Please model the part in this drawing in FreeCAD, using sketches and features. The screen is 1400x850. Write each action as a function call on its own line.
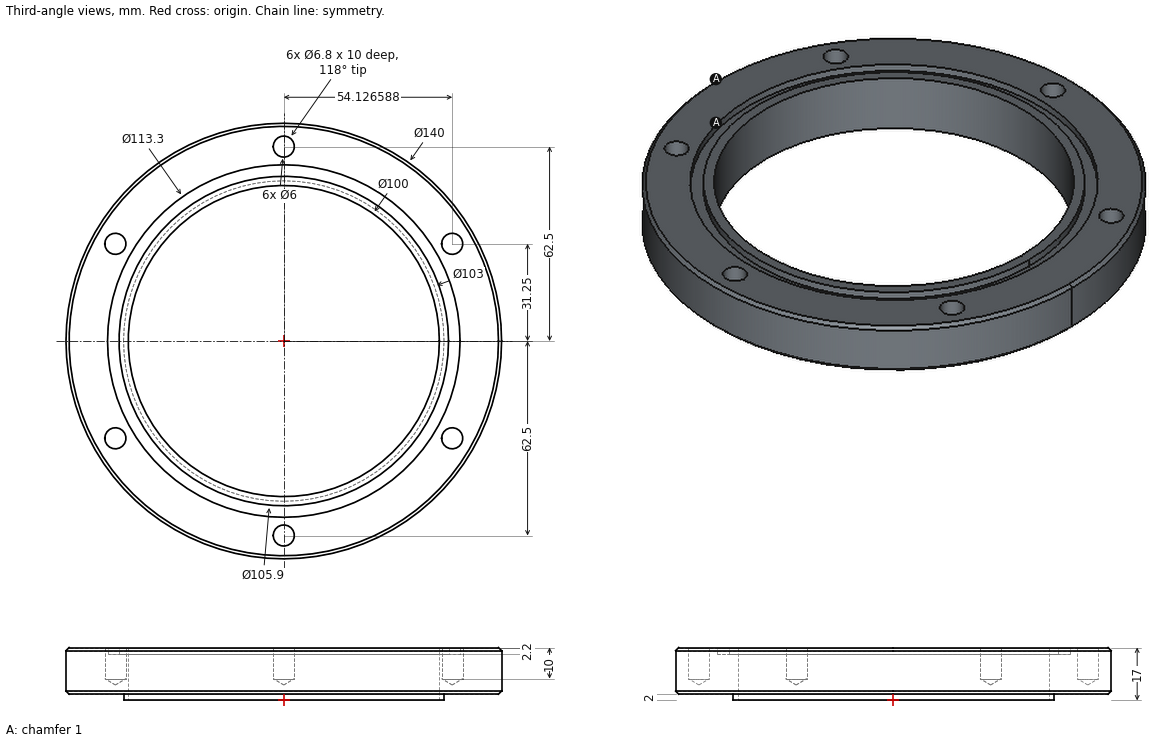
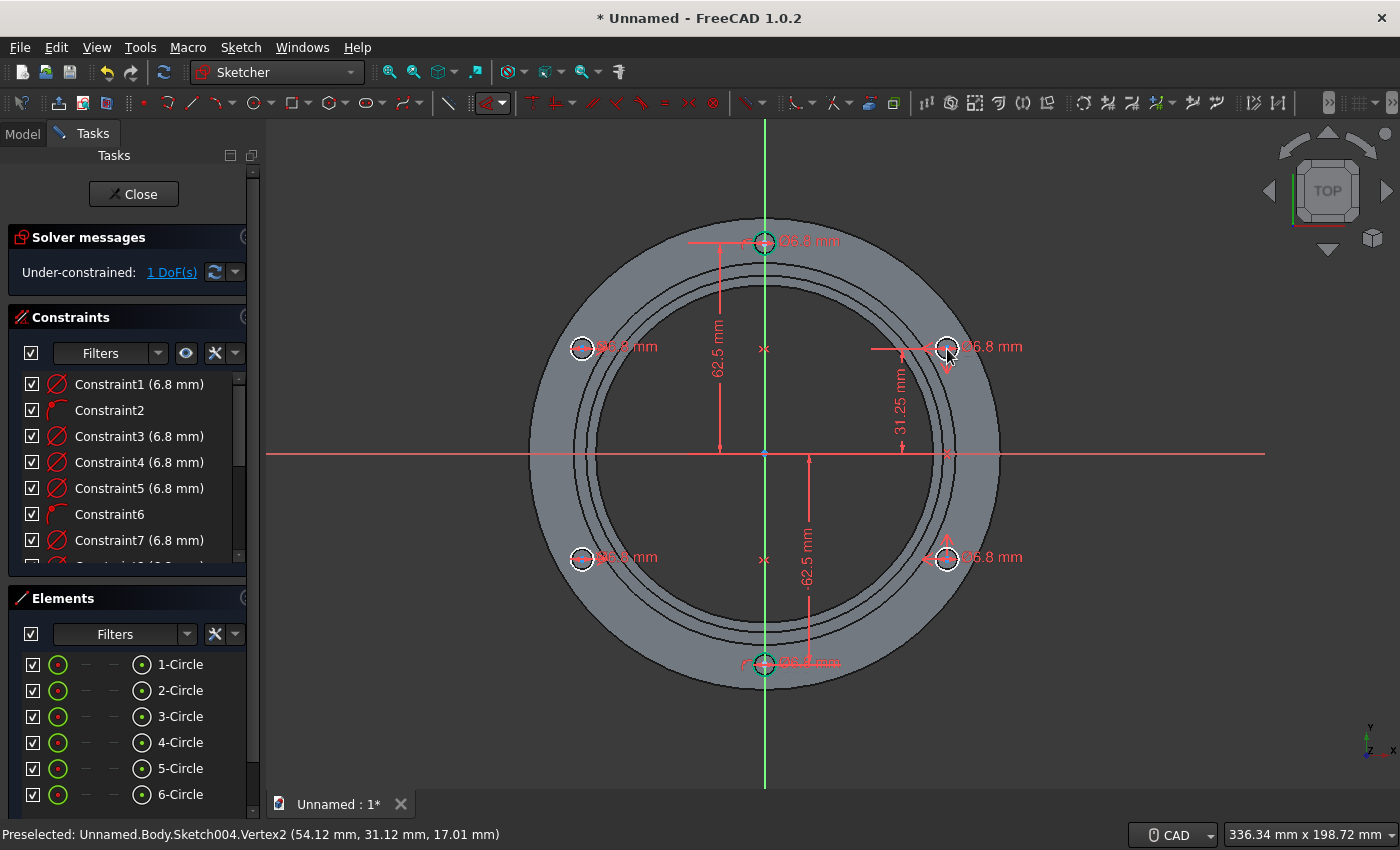
click(947, 349)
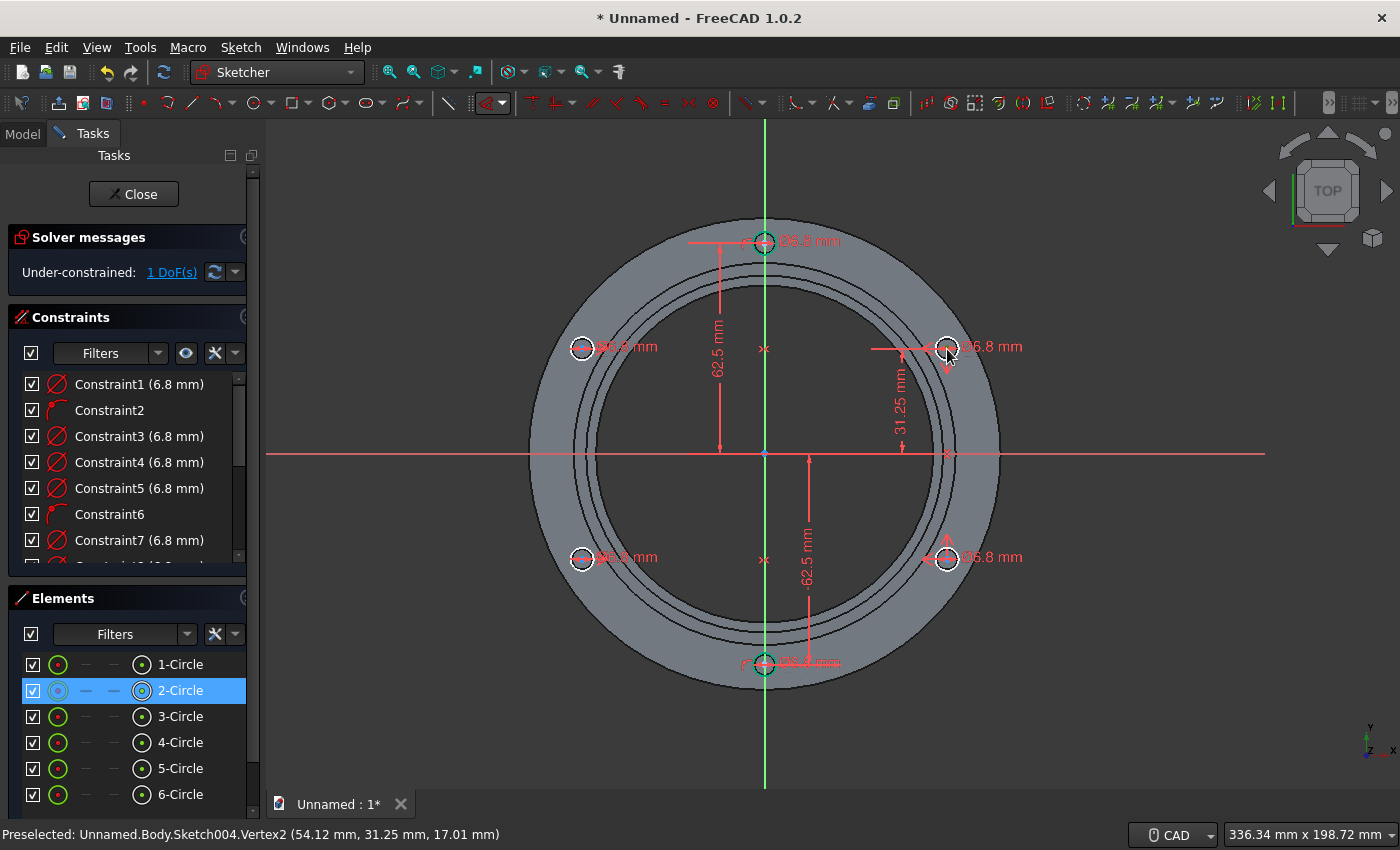
key(l)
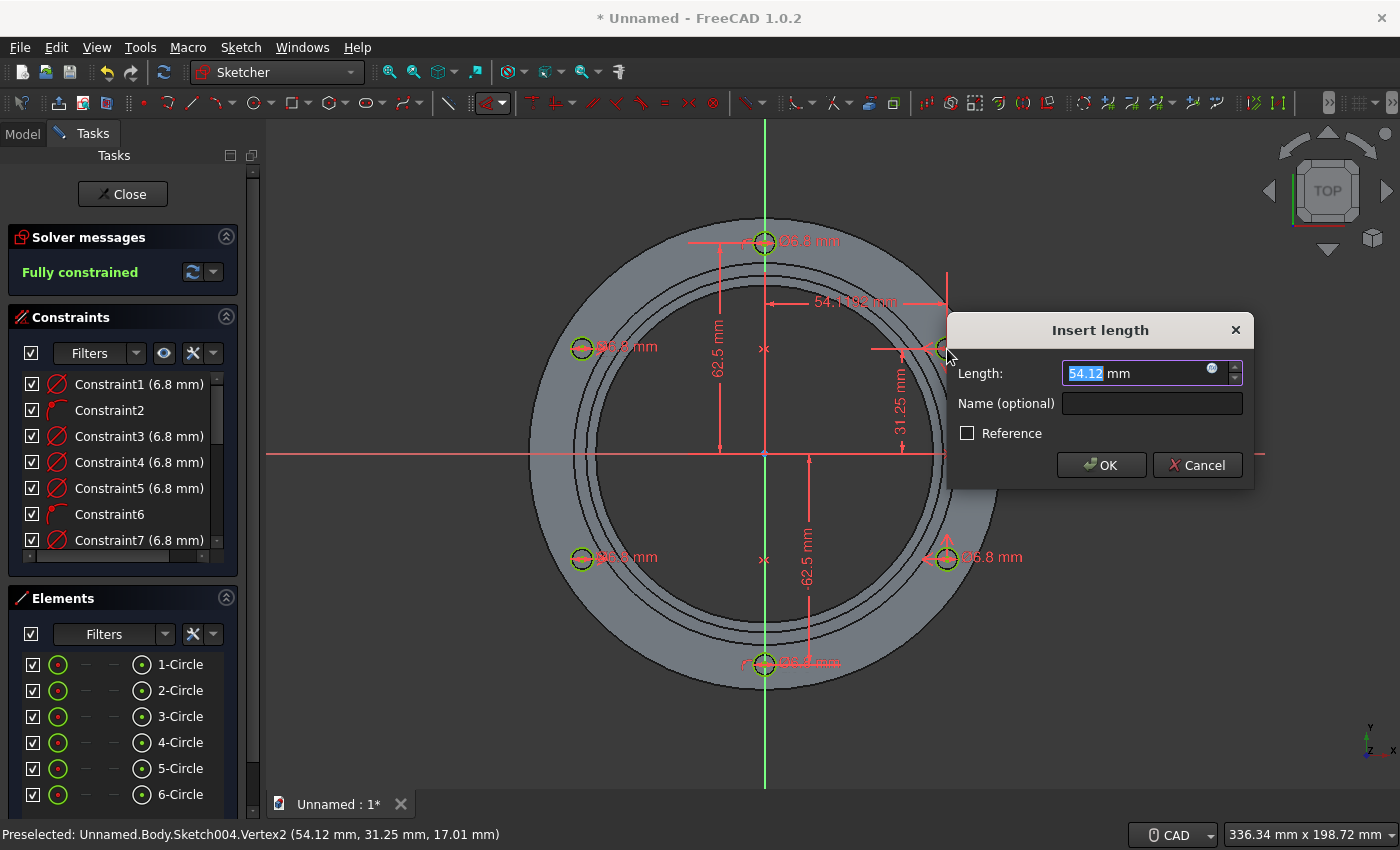
text(54.126588)
key(Return)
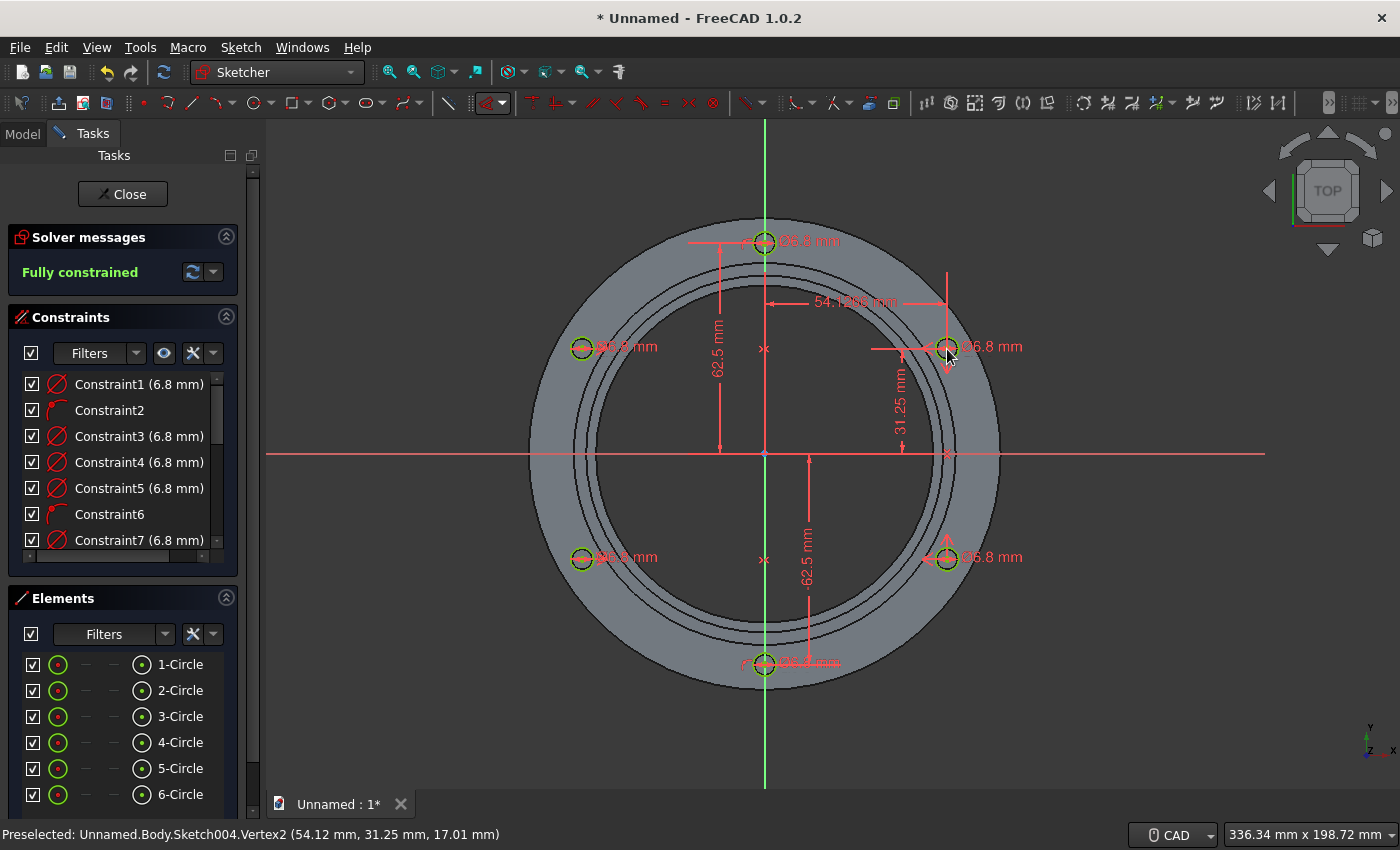
click(123, 194)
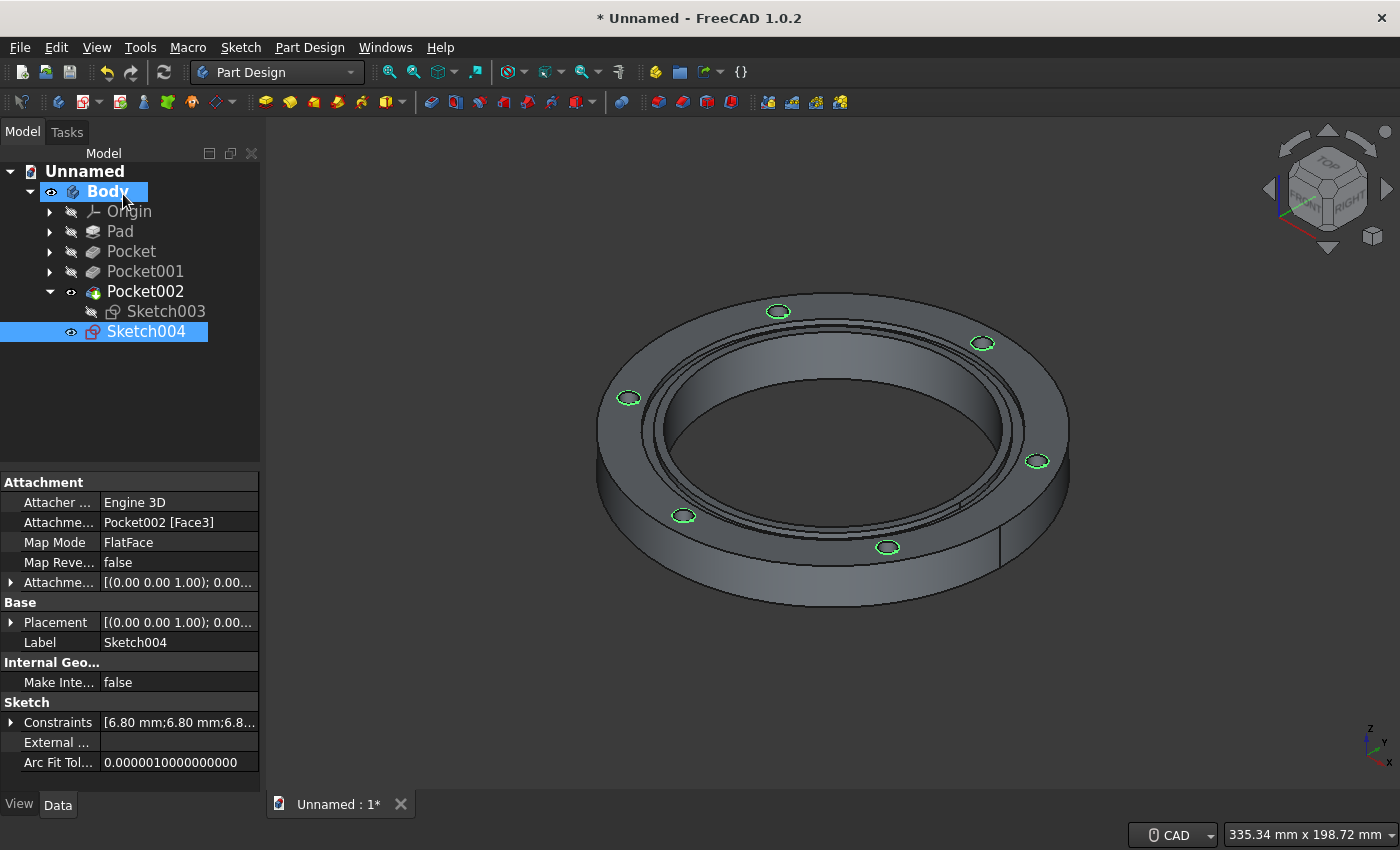
click(456, 102)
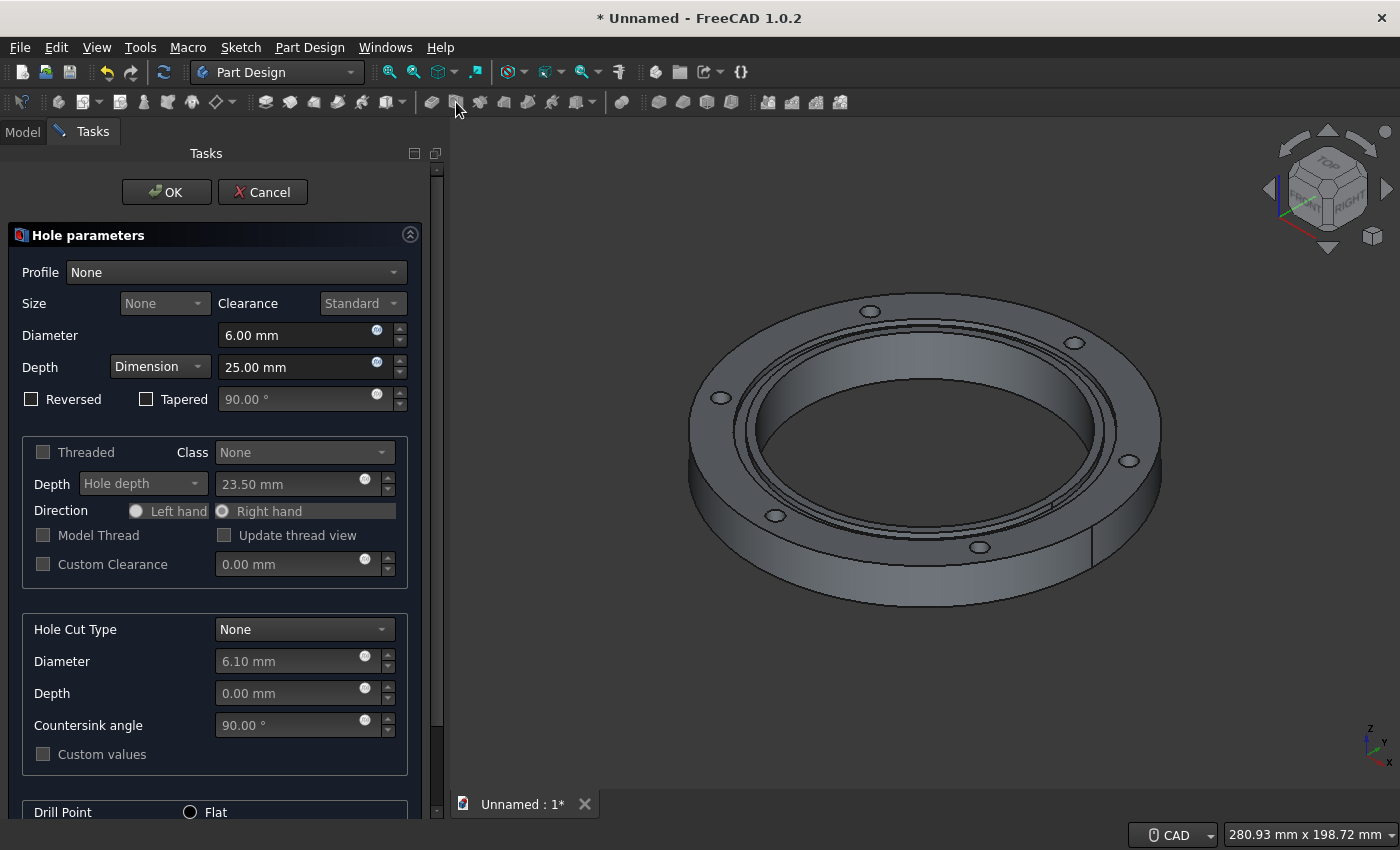
triple_click(305, 335)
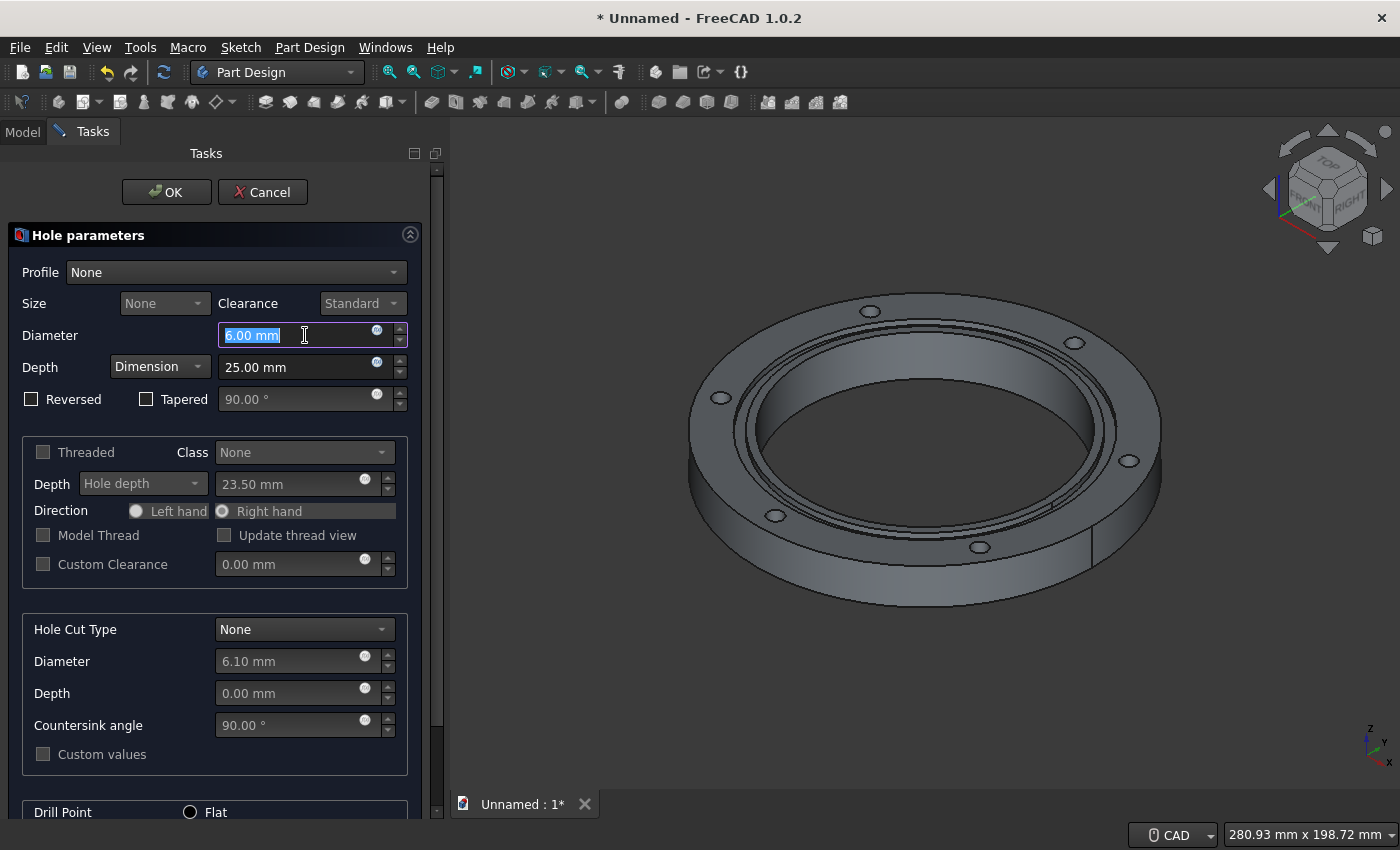
text(6.8)
key(Tab)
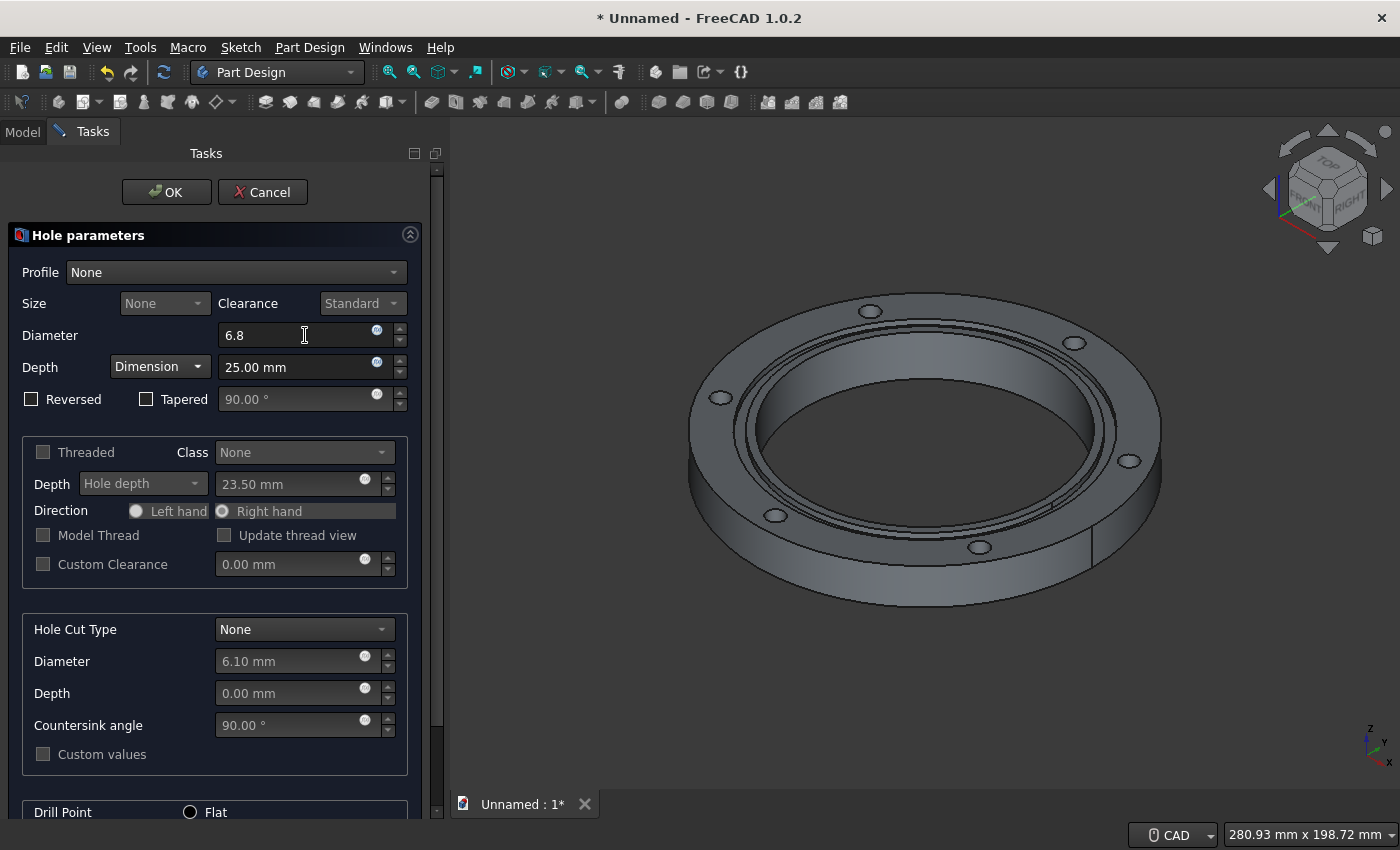
triple_click(305, 367)